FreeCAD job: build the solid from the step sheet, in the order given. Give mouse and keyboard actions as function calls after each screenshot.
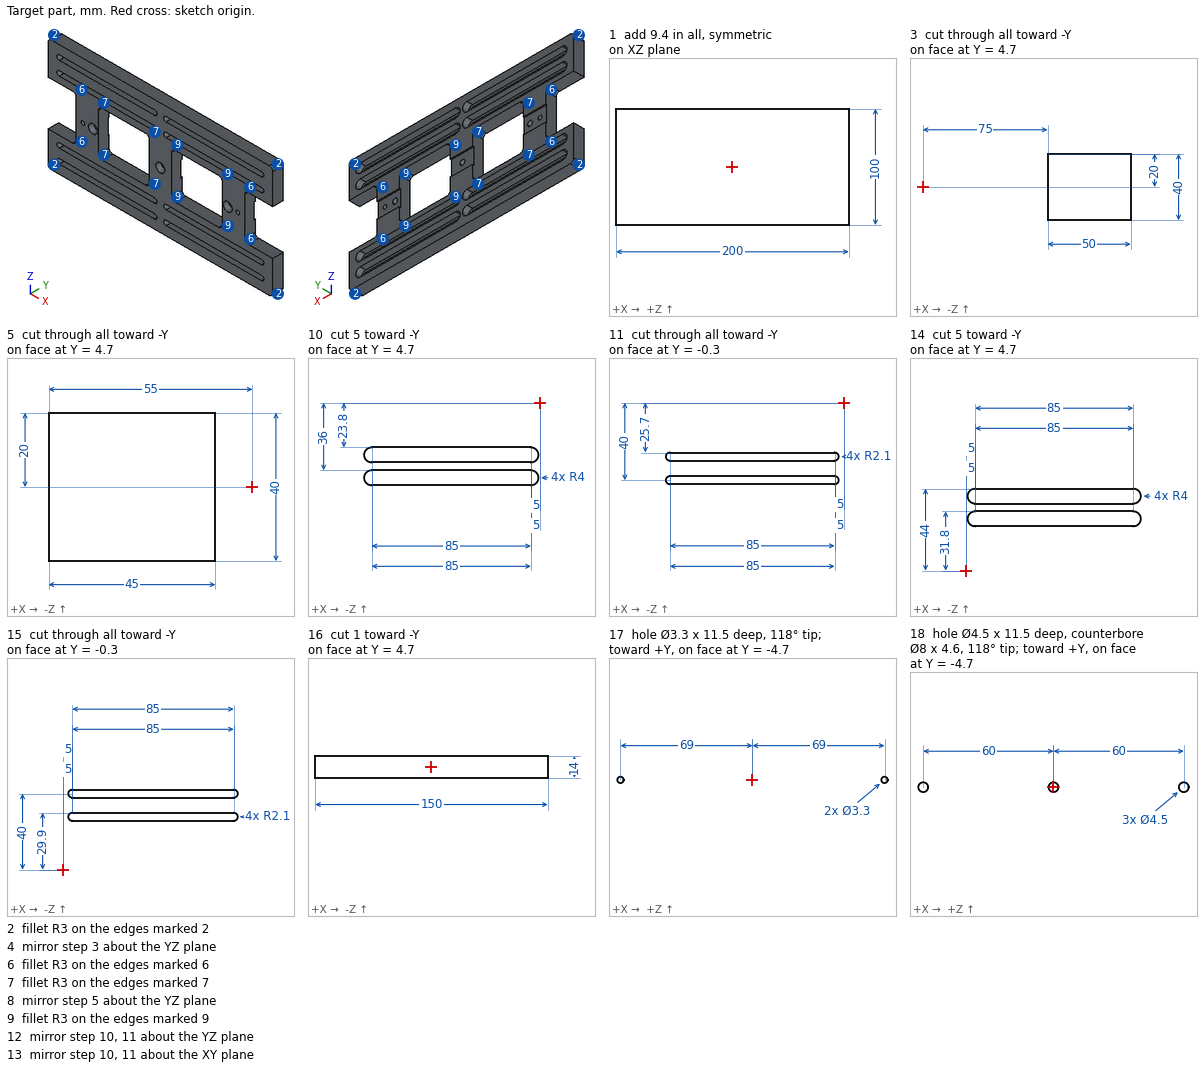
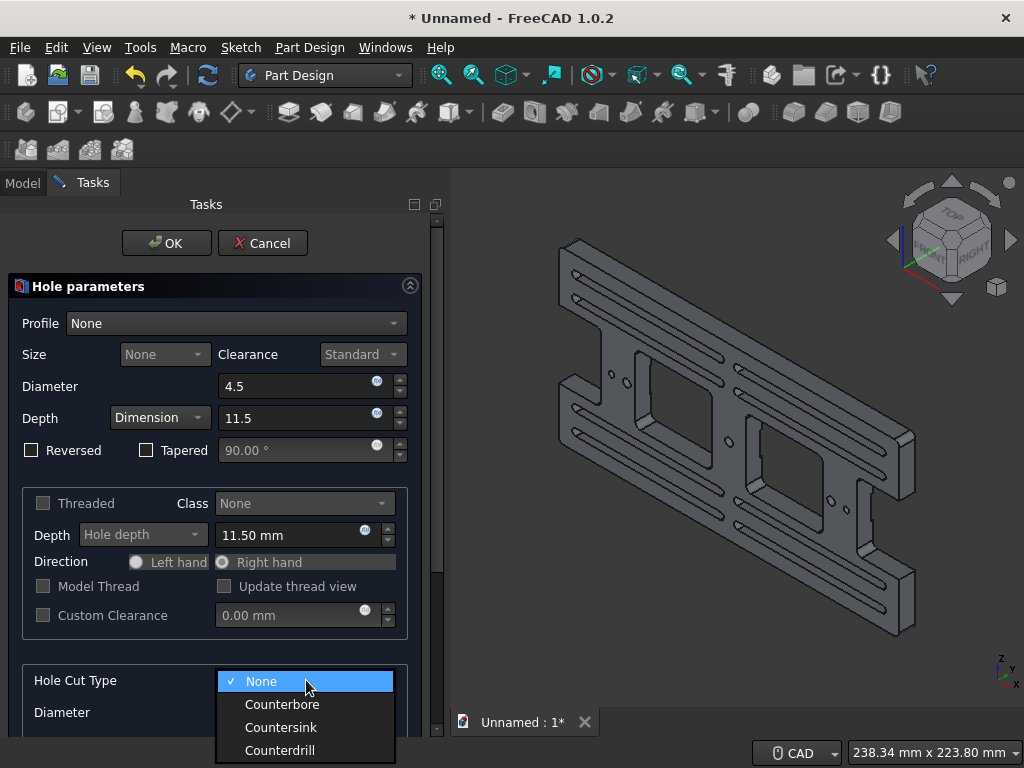
click(304, 704)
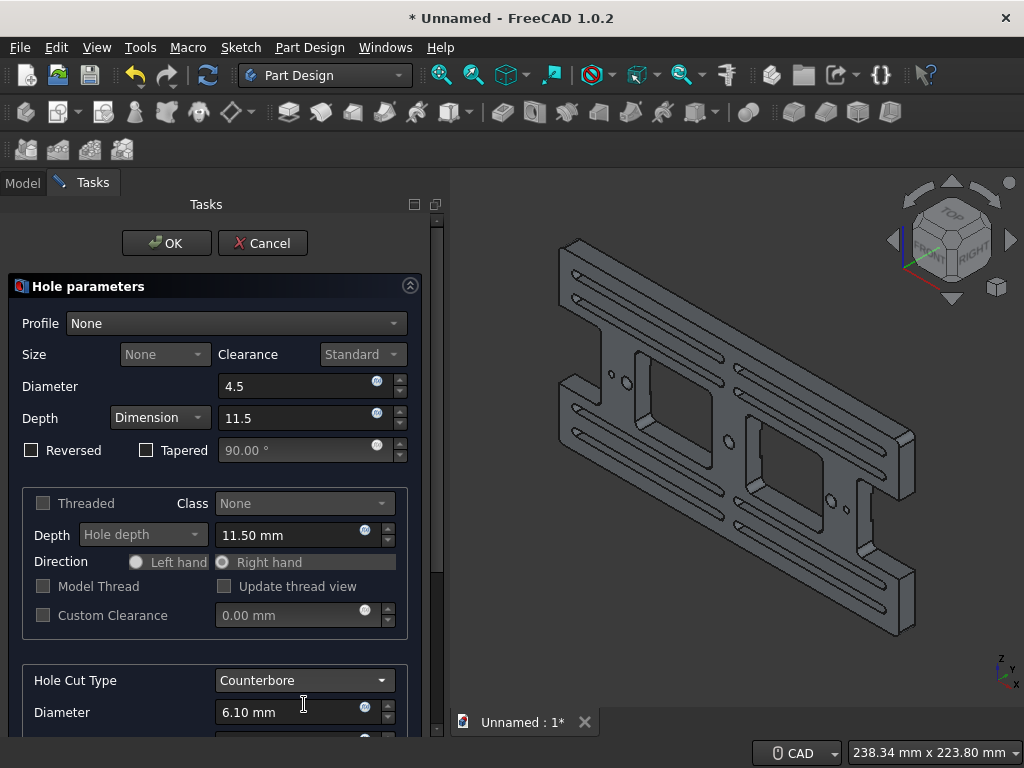
triple_click(298, 712)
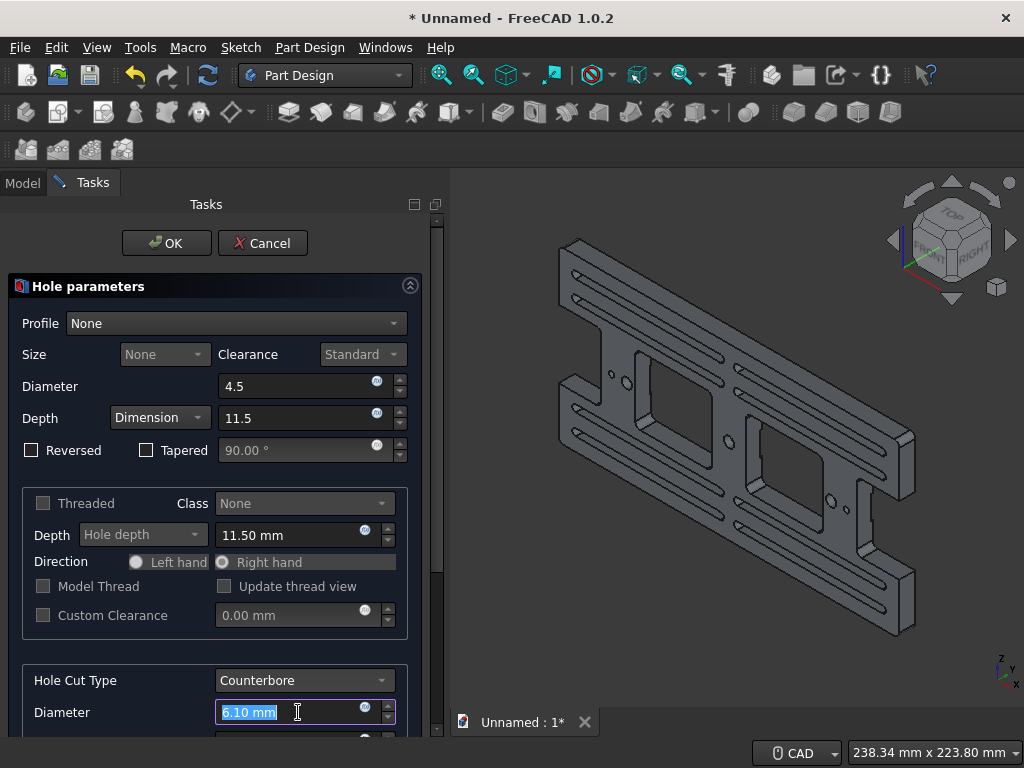
text(8)
key(Tab)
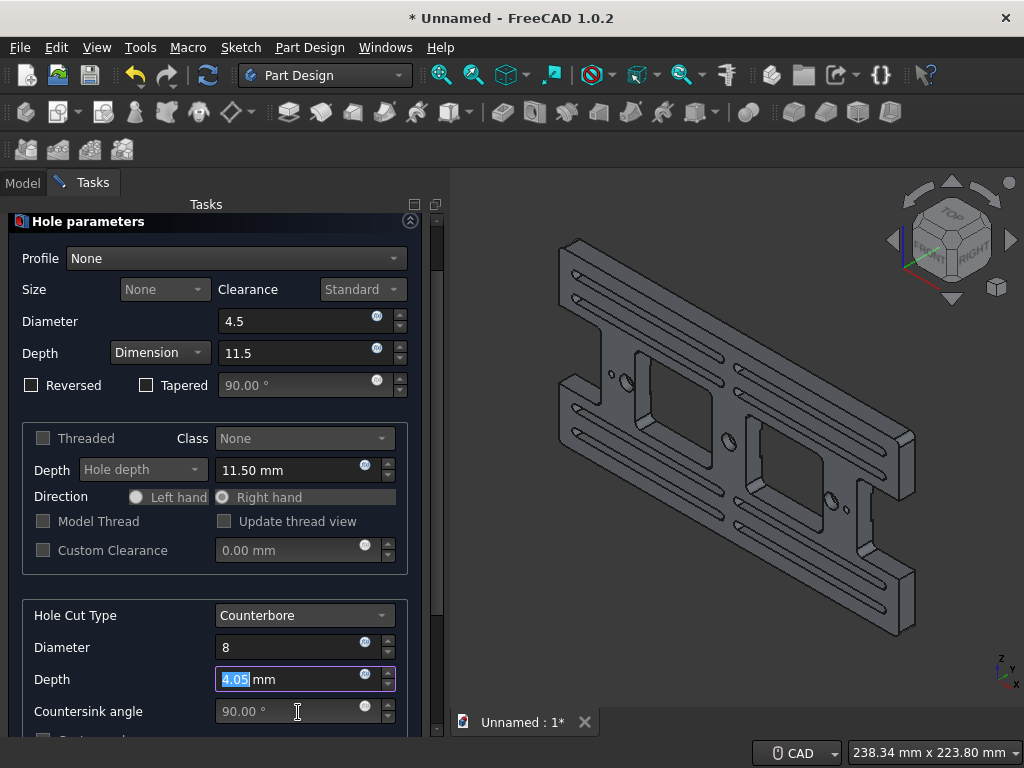
text(4.6)
key(Tab)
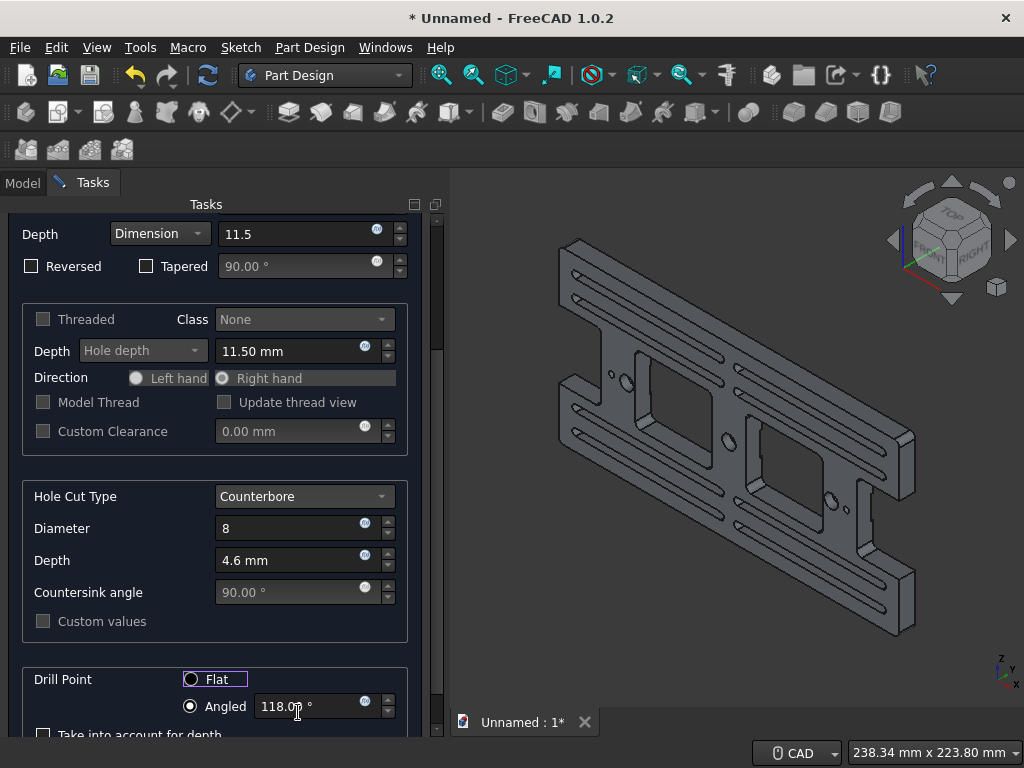
scroll(437, 475, up, 4)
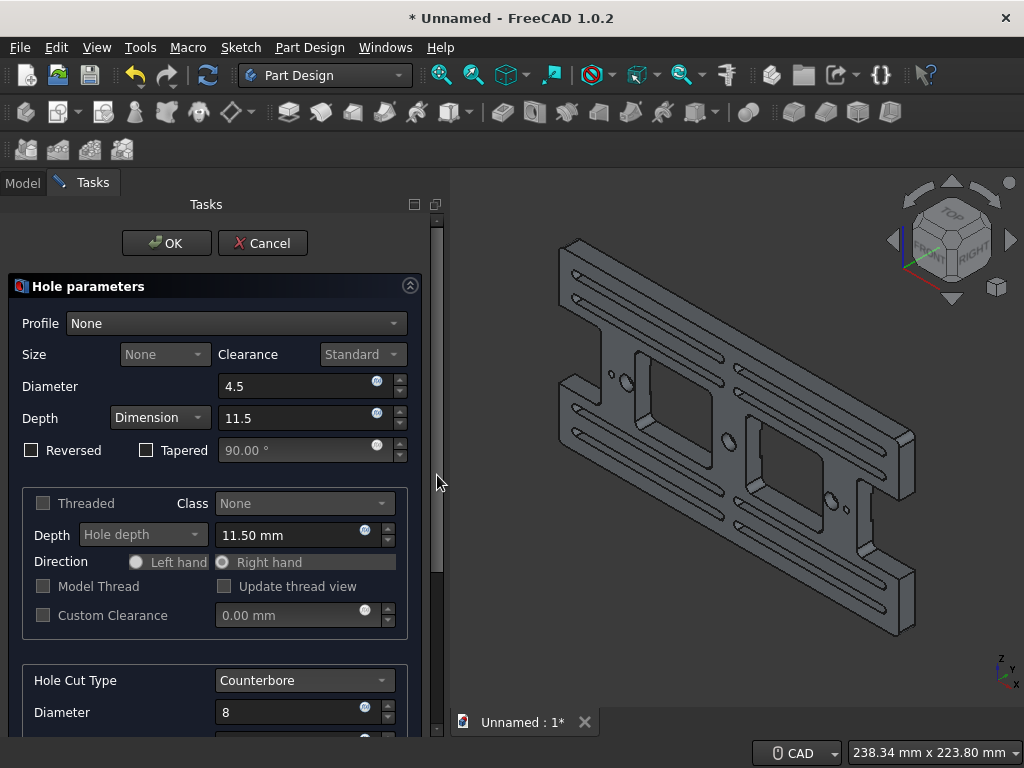
click(167, 243)